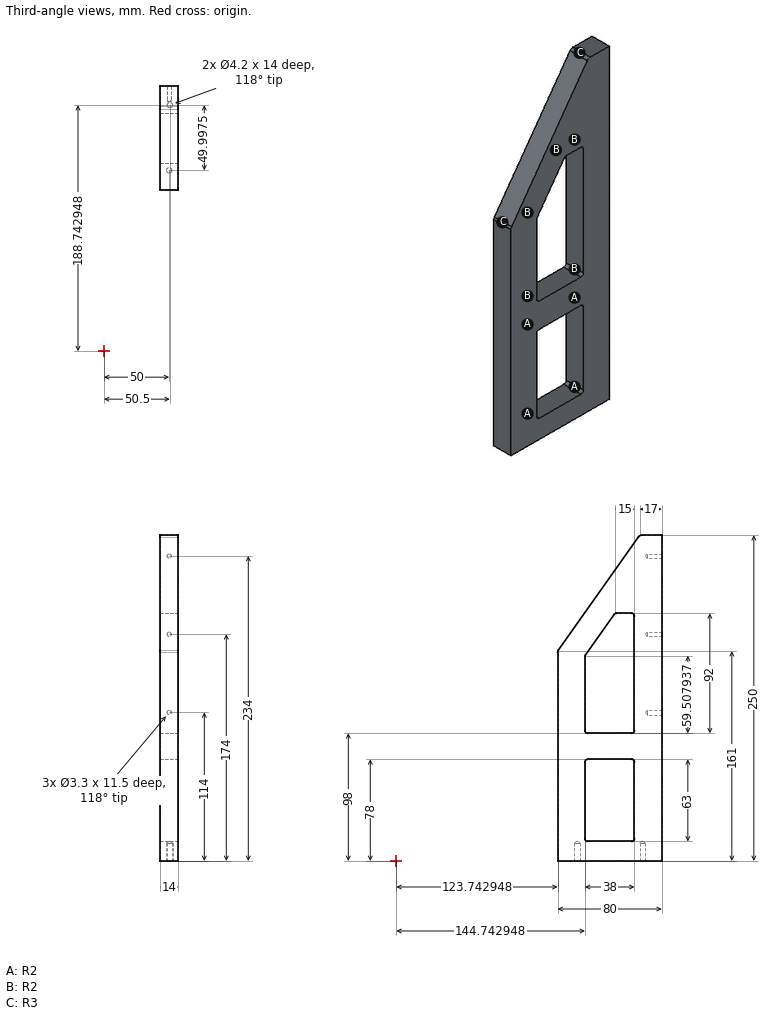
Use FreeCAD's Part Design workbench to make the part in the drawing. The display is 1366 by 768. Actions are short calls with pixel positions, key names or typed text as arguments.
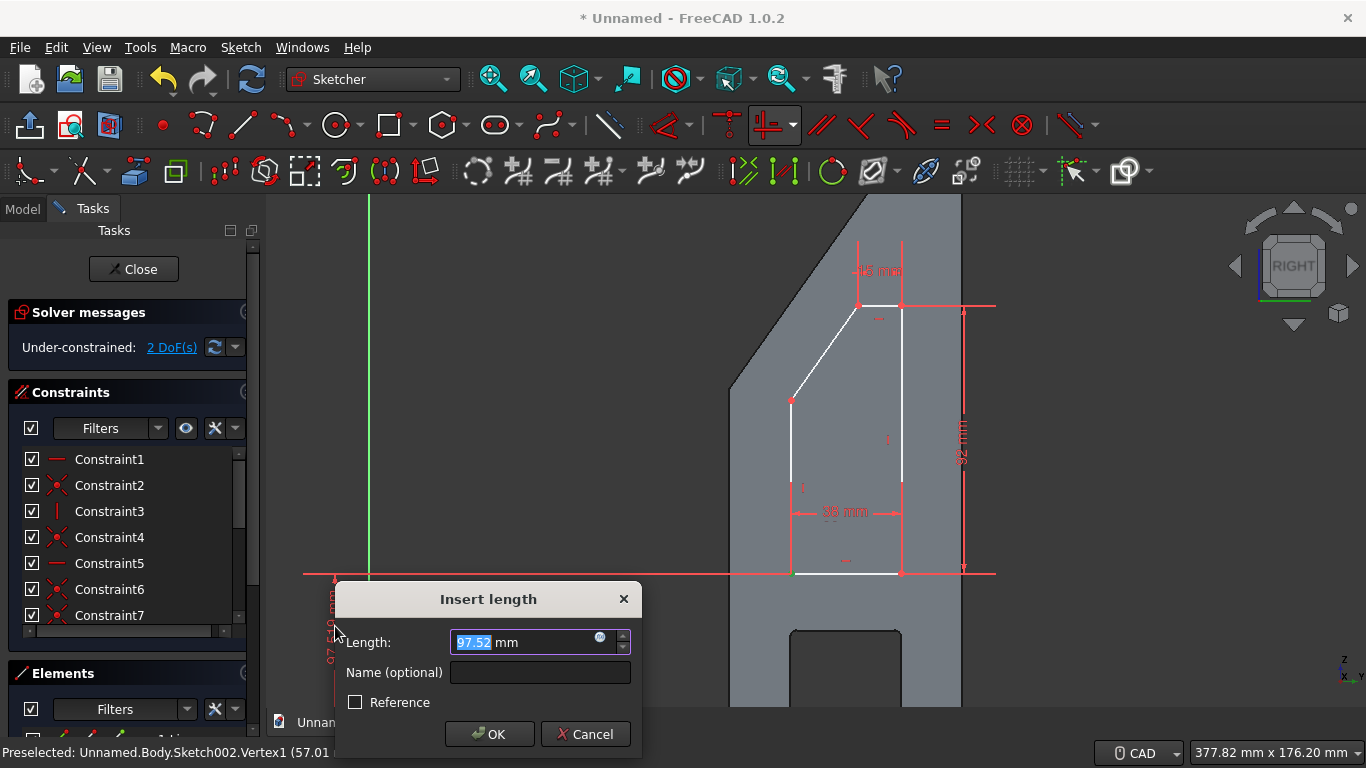
text(98)
key(Return)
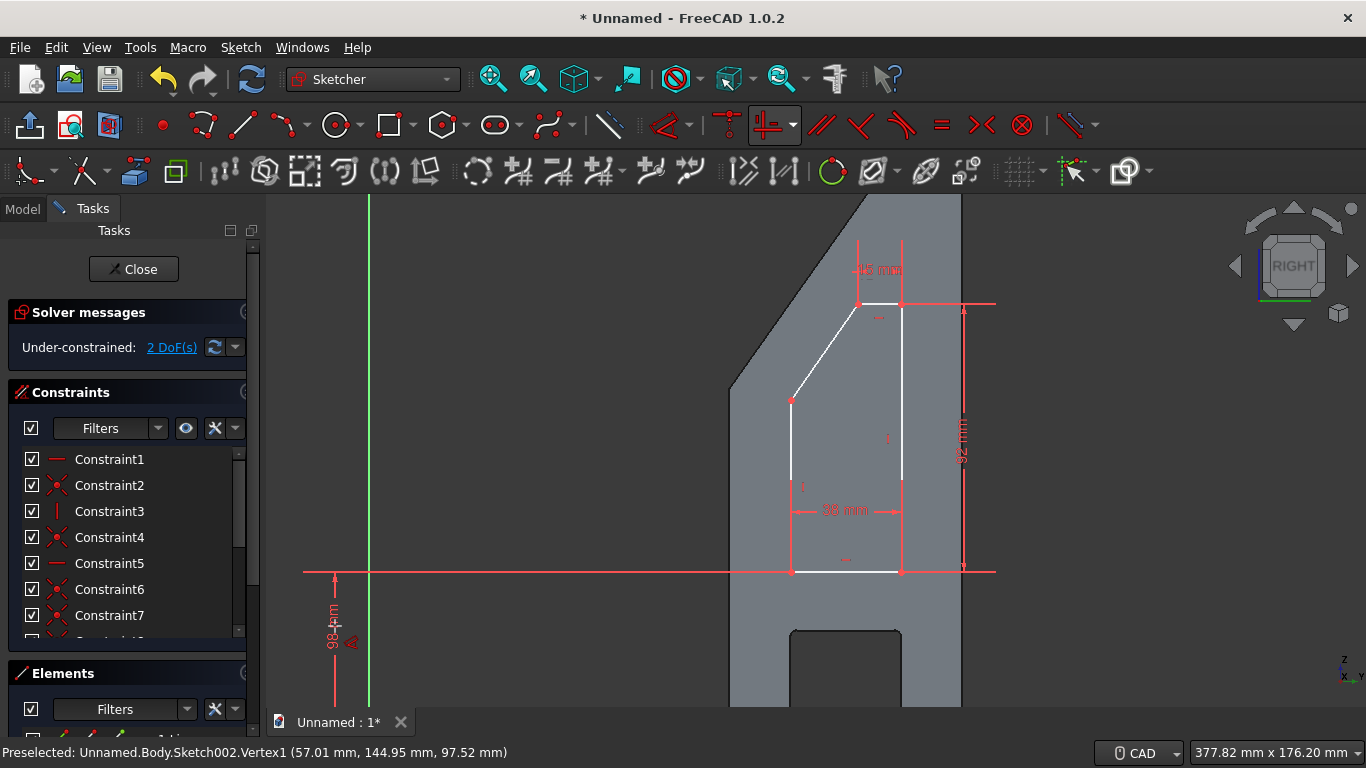
click(791, 452)
click(825, 486)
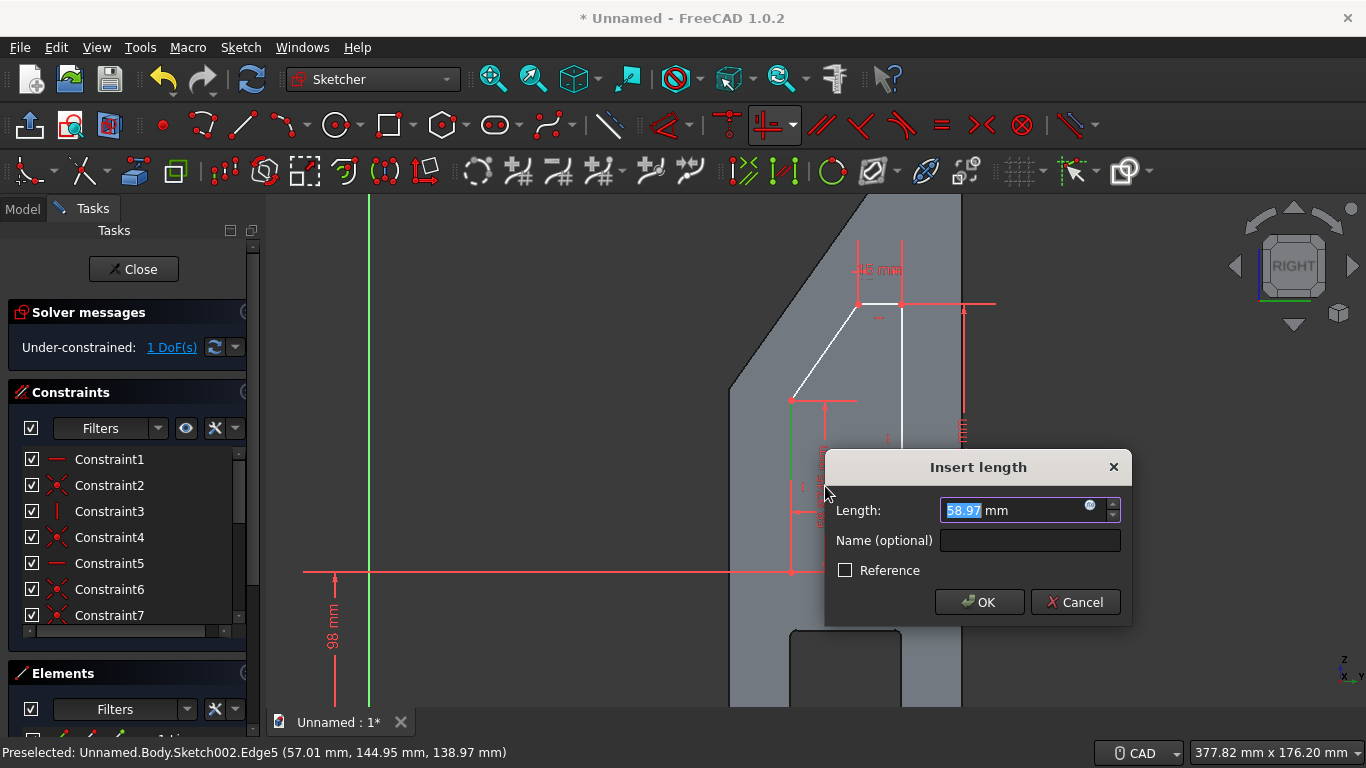
text(59.507937)
key(Return)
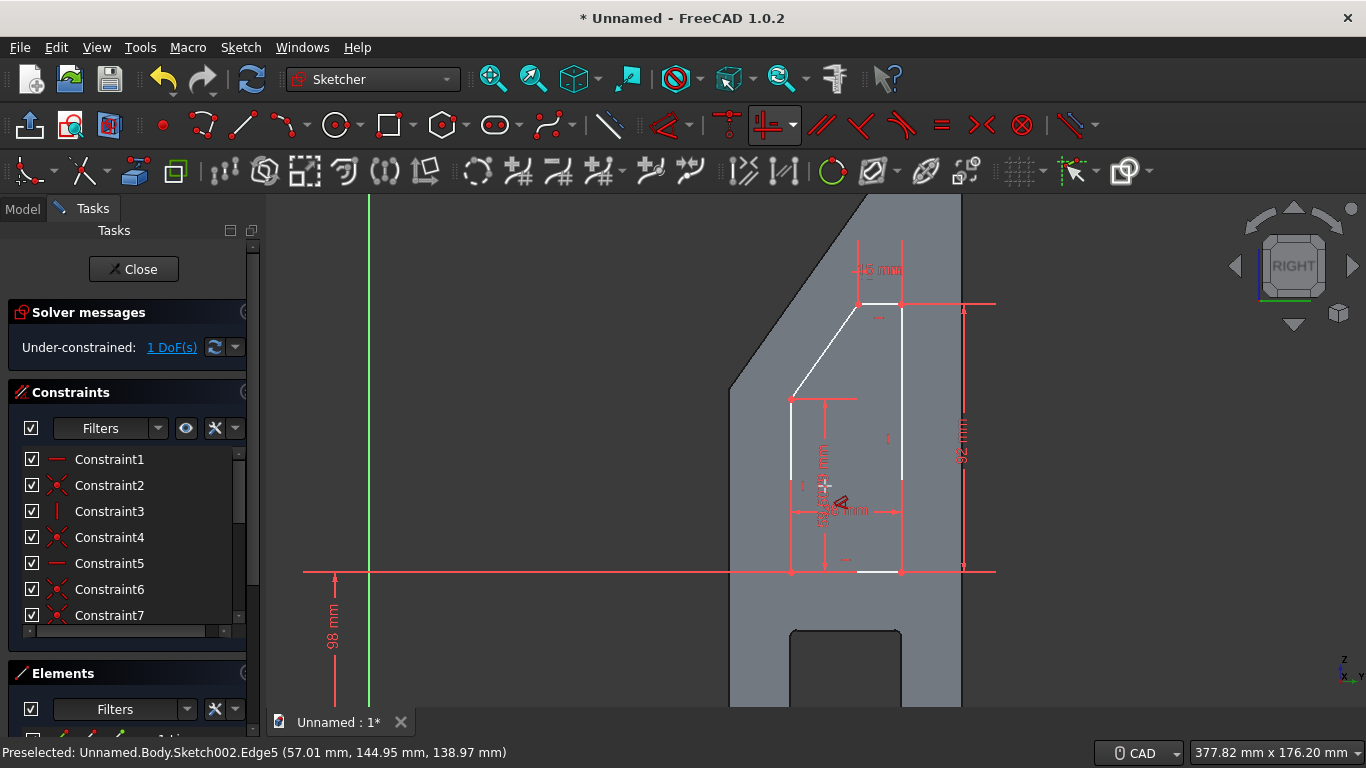
click(791, 572)
click(580, 538)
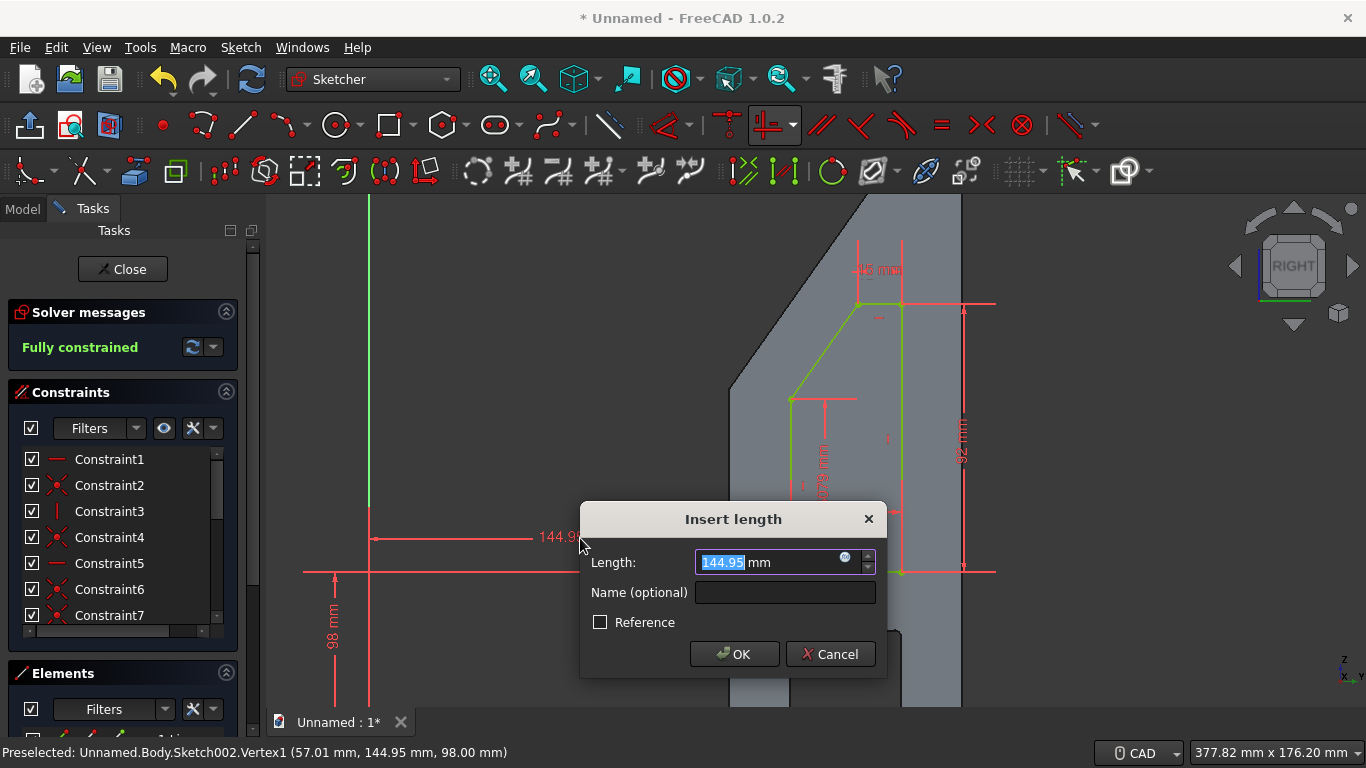
text(144.742948)
key(Return)
key(Escape)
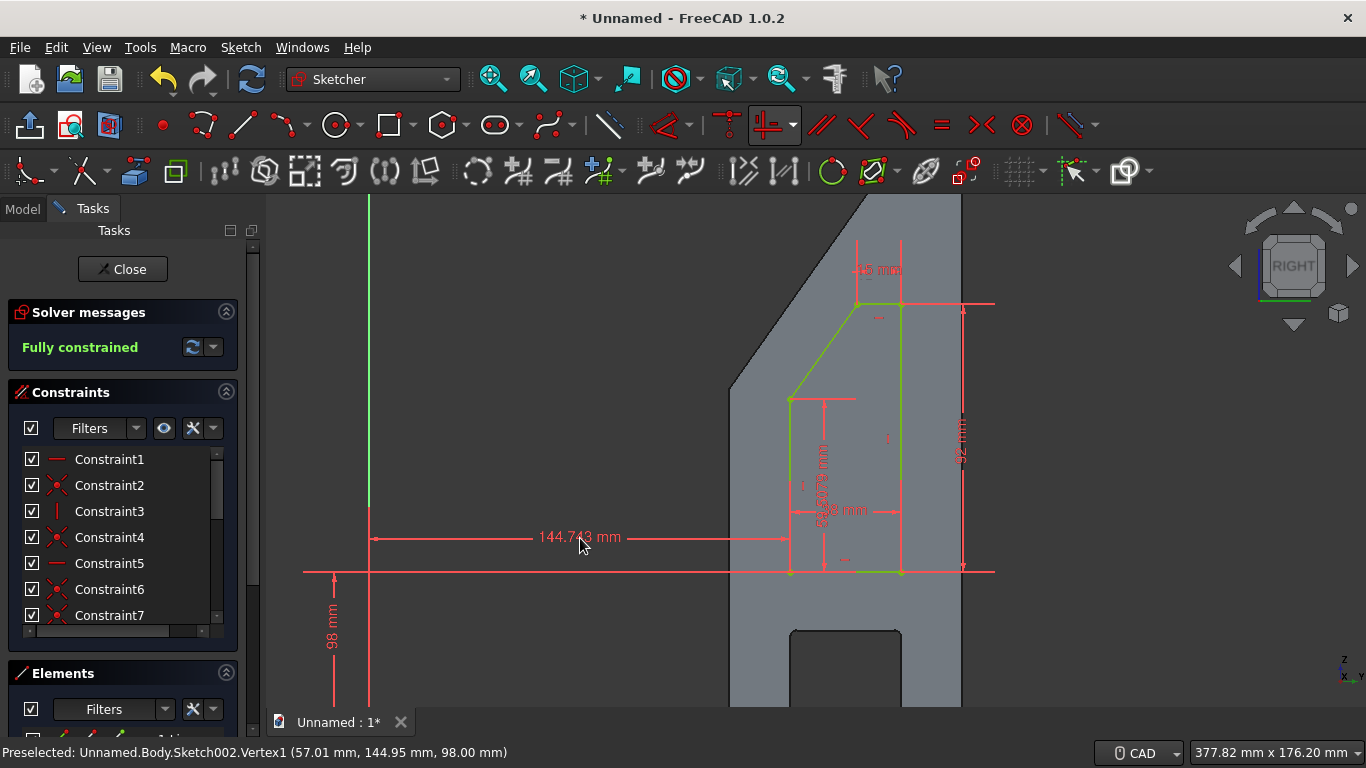
click(123, 269)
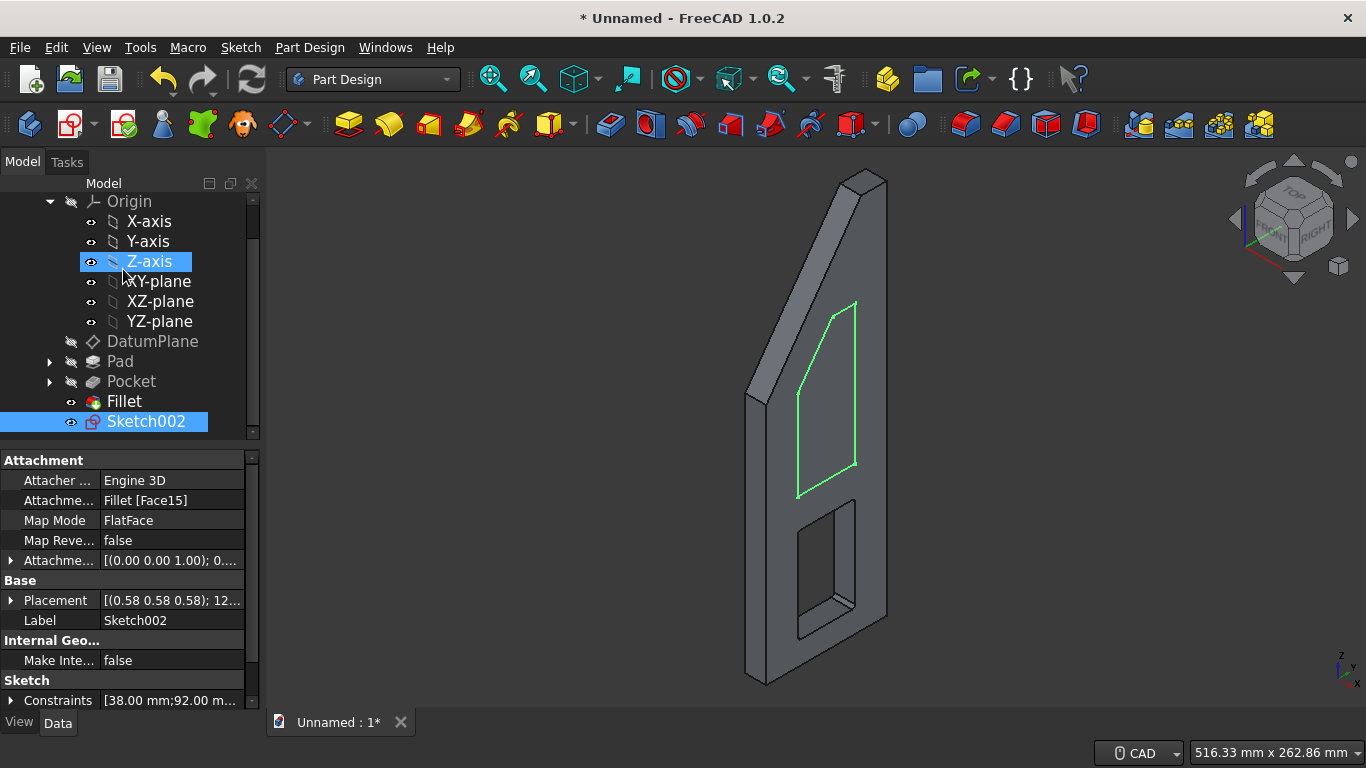
click(612, 124)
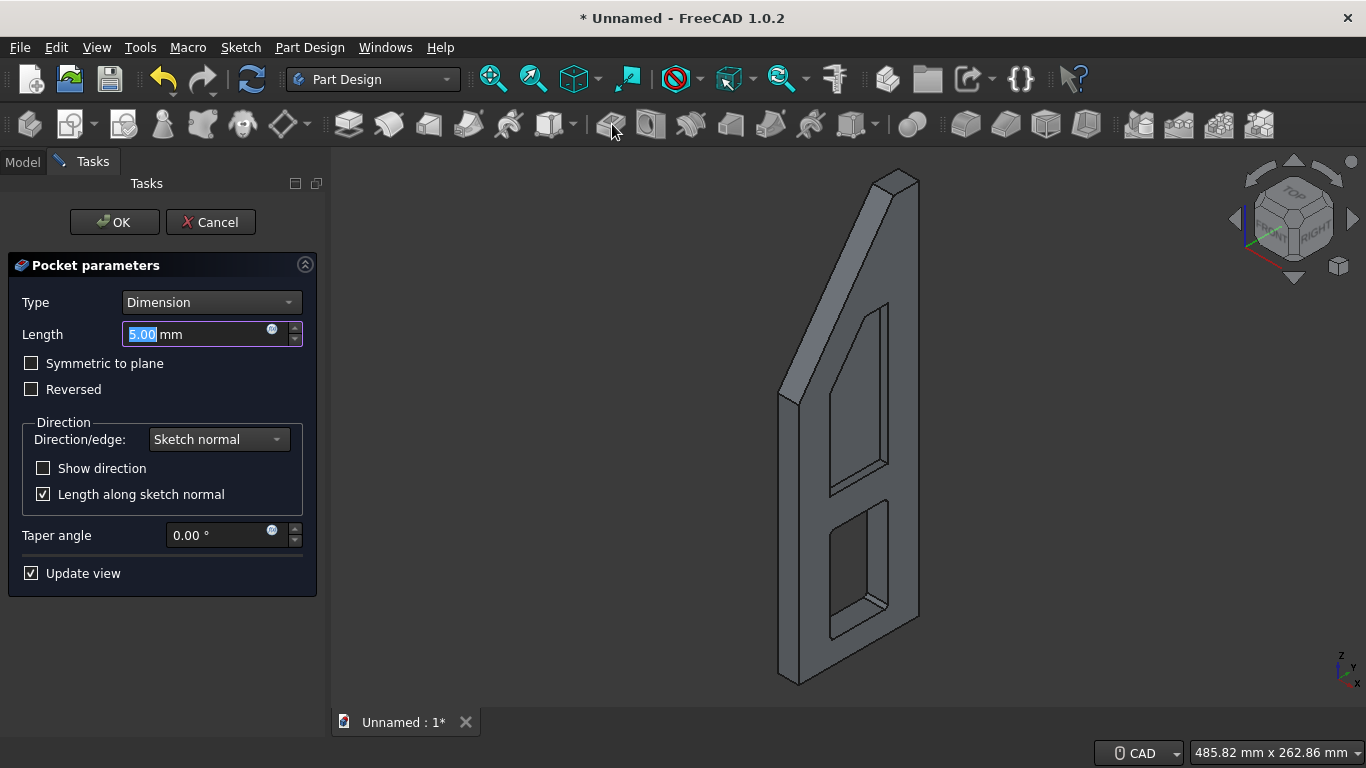
click(212, 302)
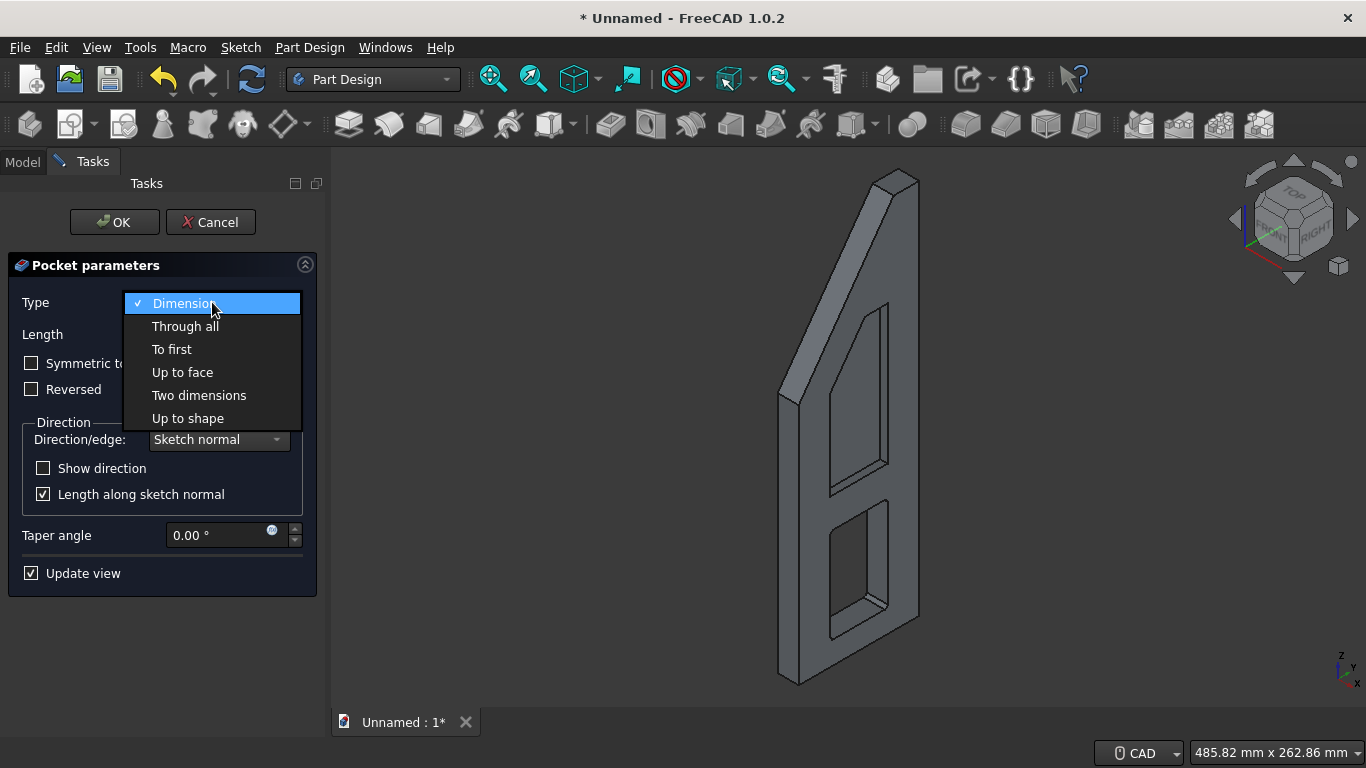
click(212, 326)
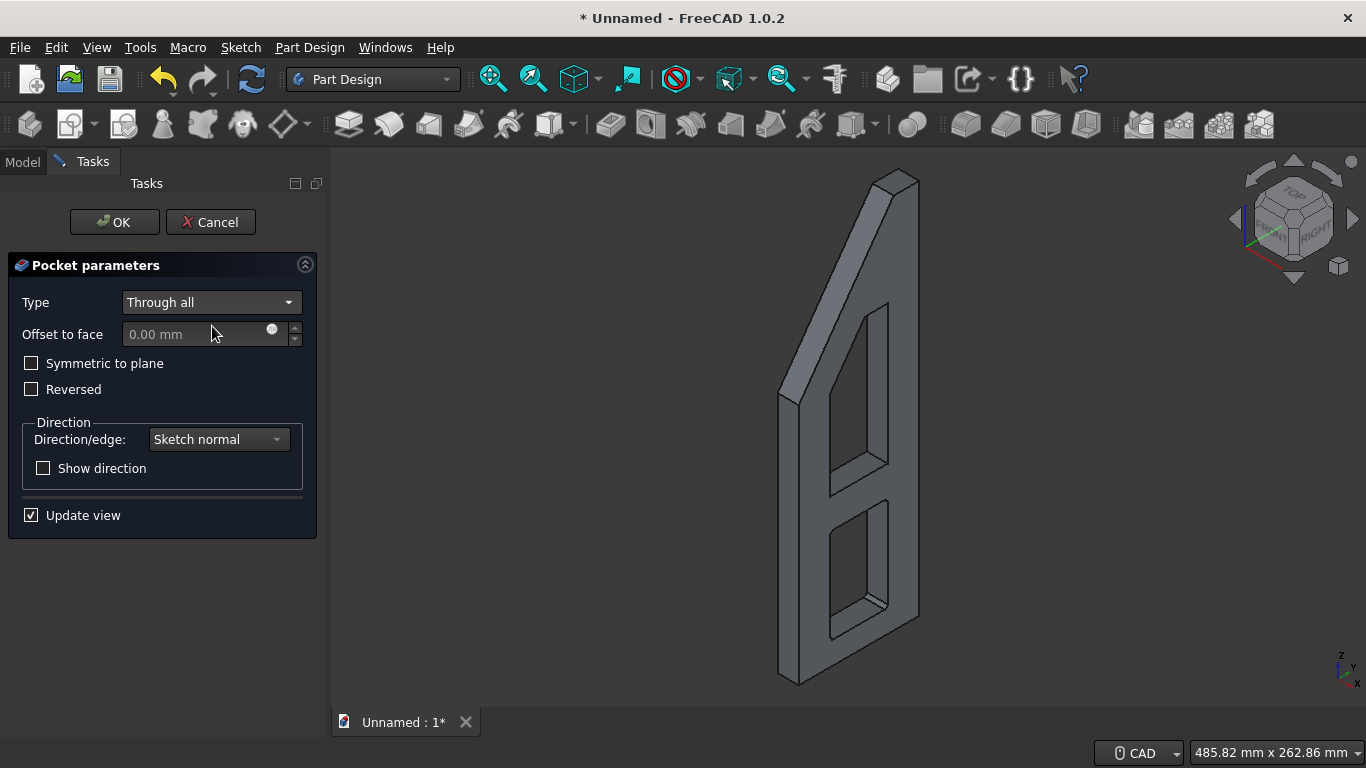
click(115, 222)